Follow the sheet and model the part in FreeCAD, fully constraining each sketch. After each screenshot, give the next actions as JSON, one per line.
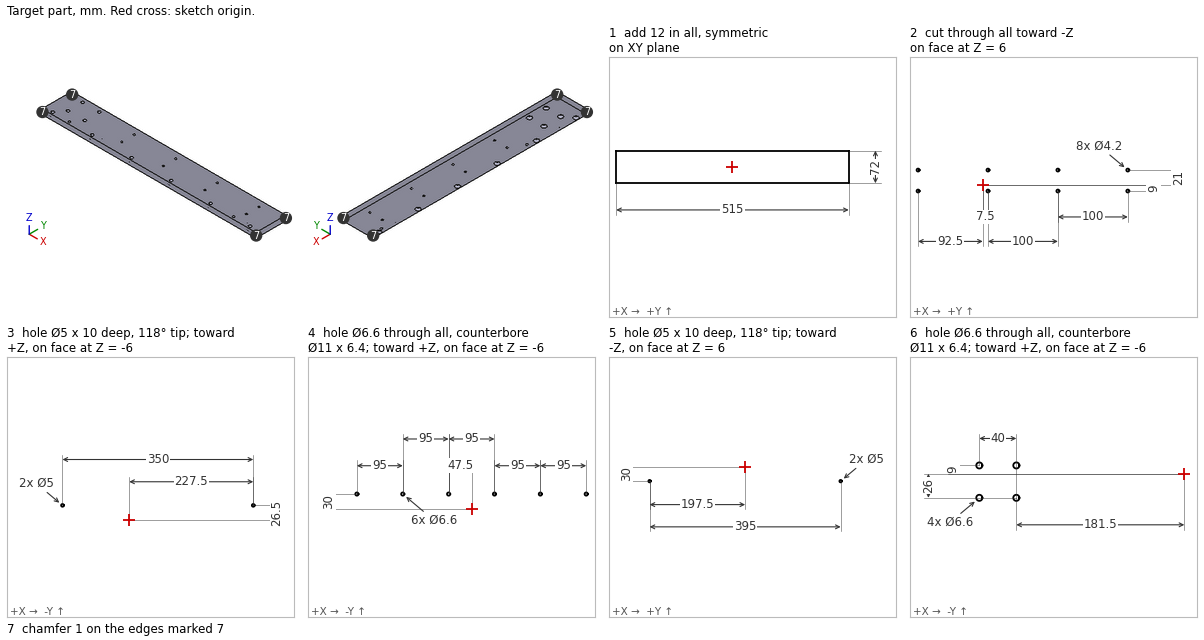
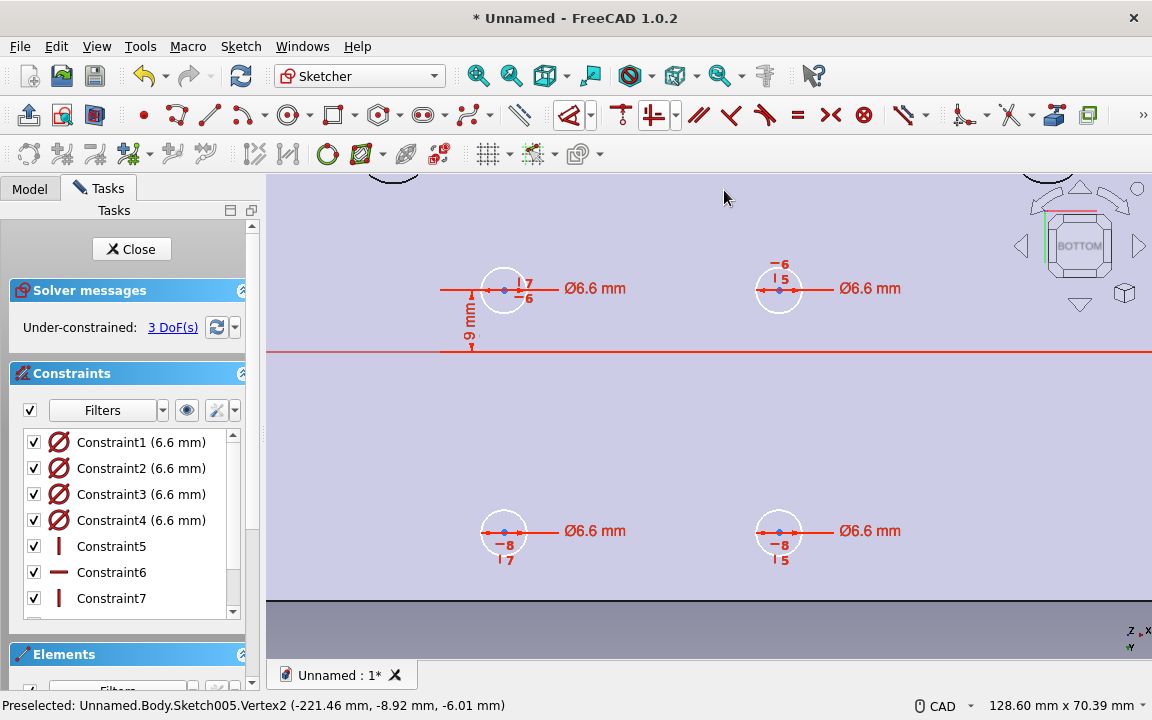
{"action": "left_click", "coordinate": [779, 533]}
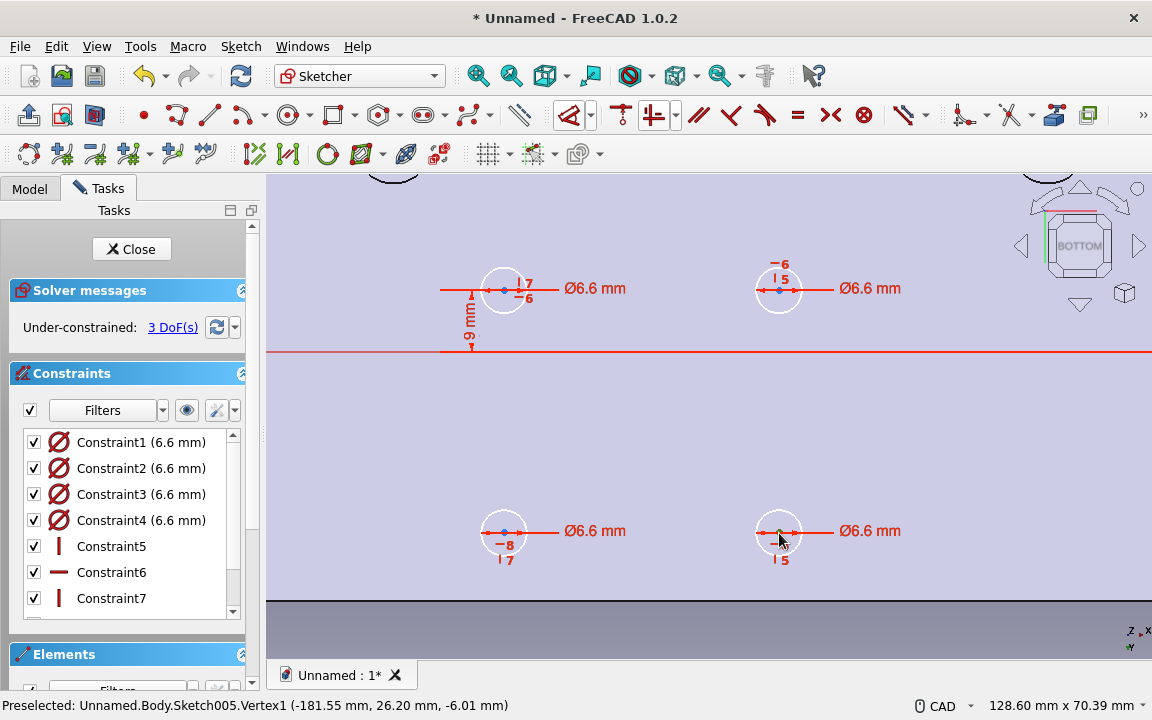
{"action": "left_click", "coordinate": [590, 116]}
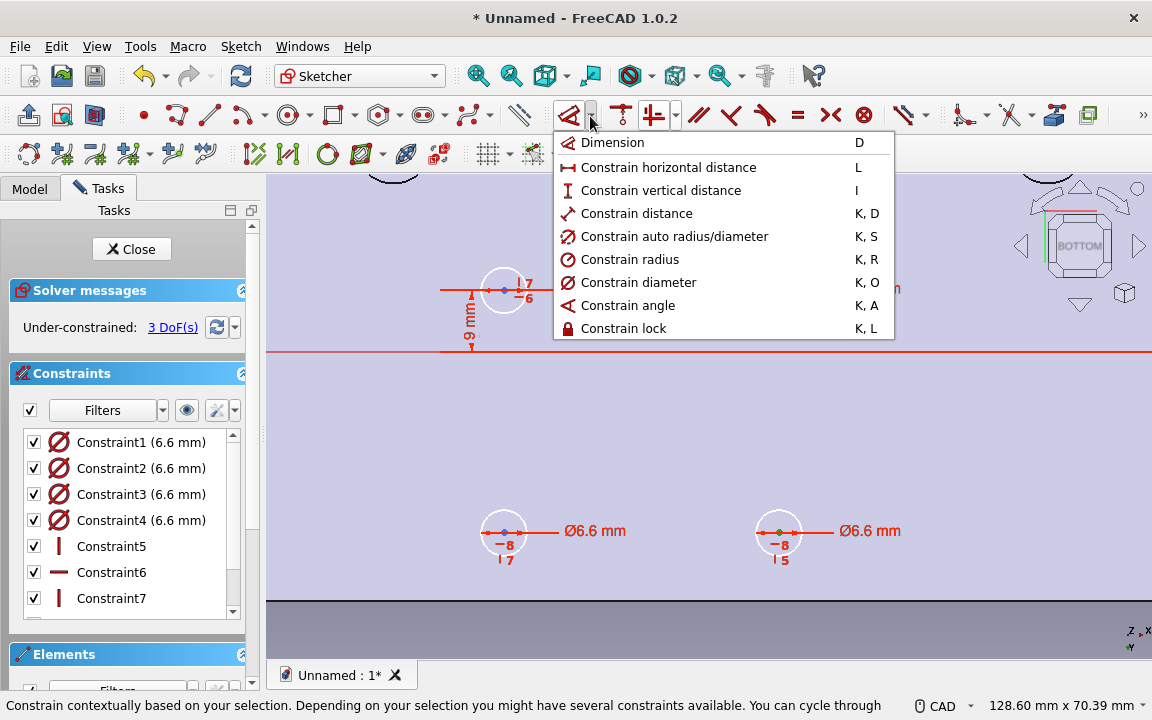
{"action": "left_click", "coordinate": [724, 190]}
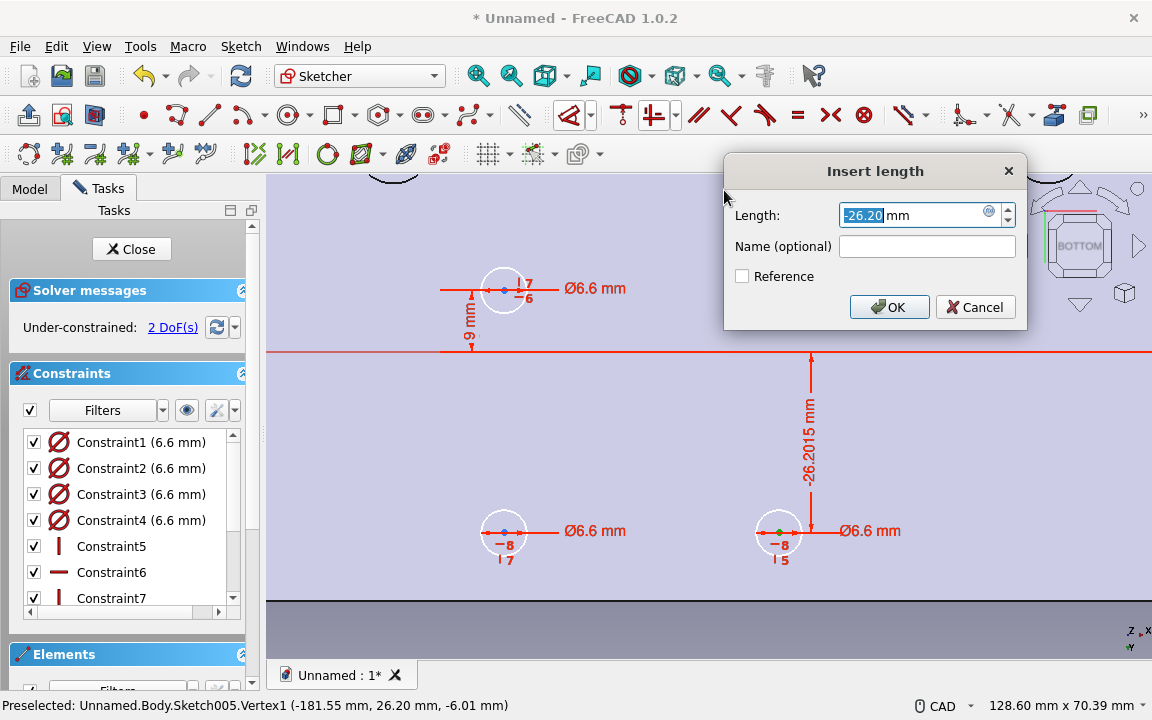
{"action": "type", "text": "-26"}
{"action": "key", "text": "Return"}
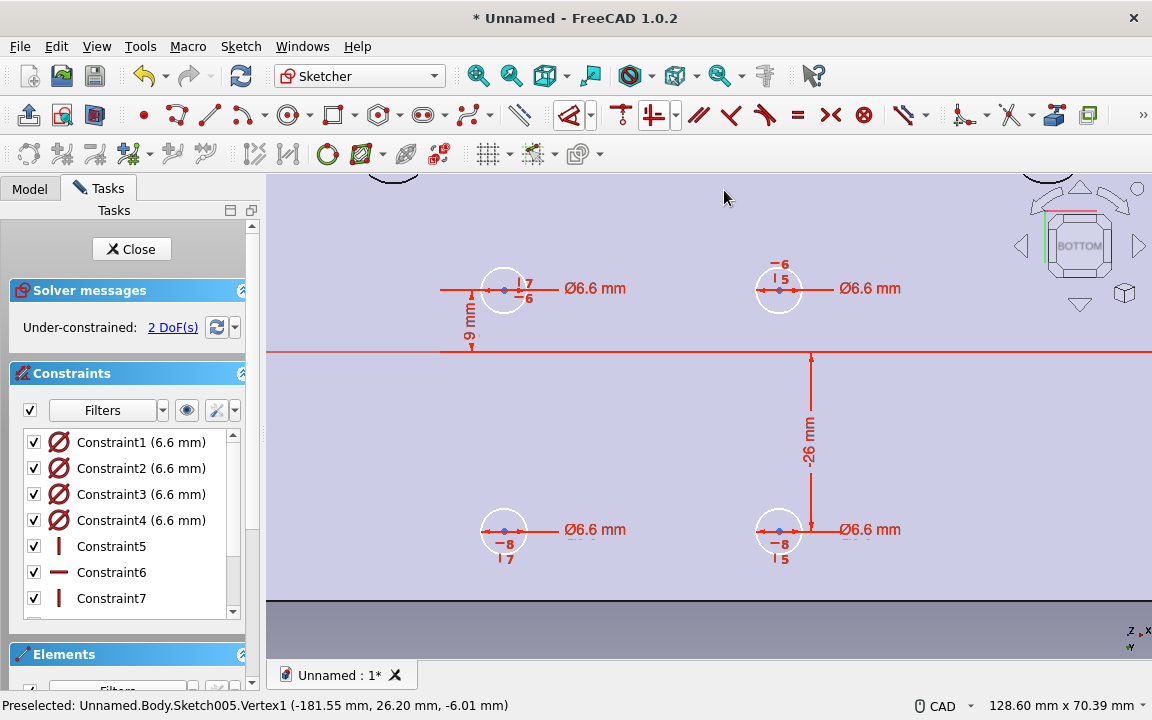
{"action": "left_click", "coordinate": [779, 532]}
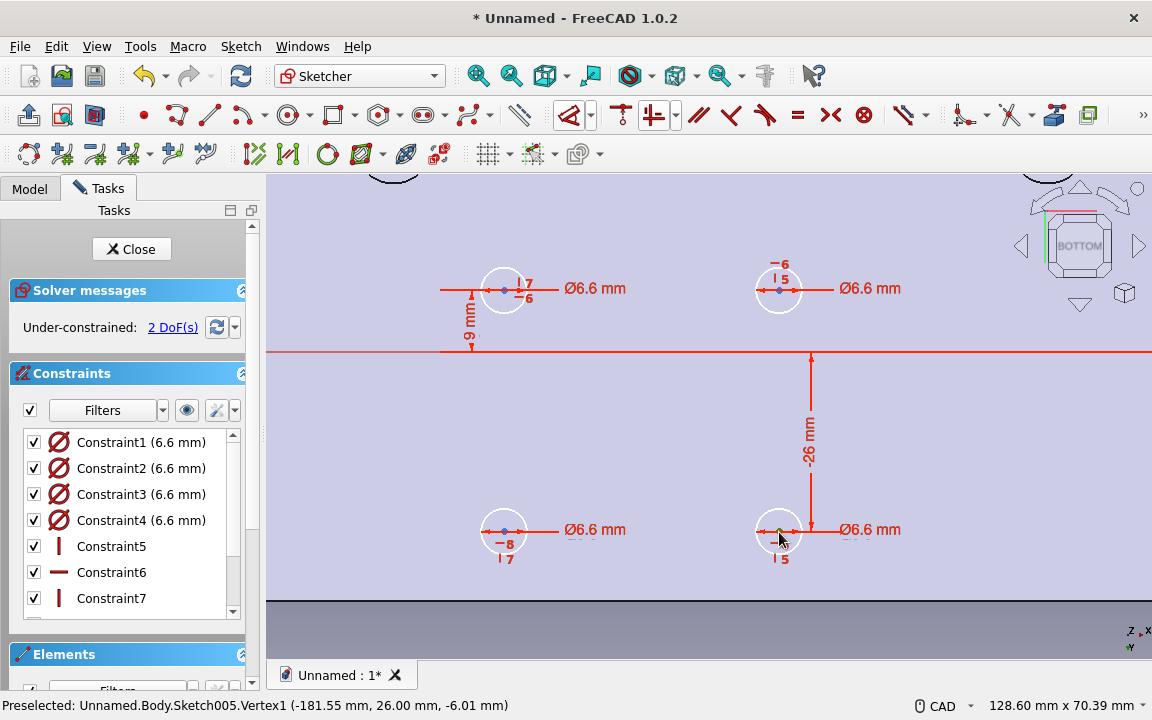
{"action": "left_click", "coordinate": [504, 290]}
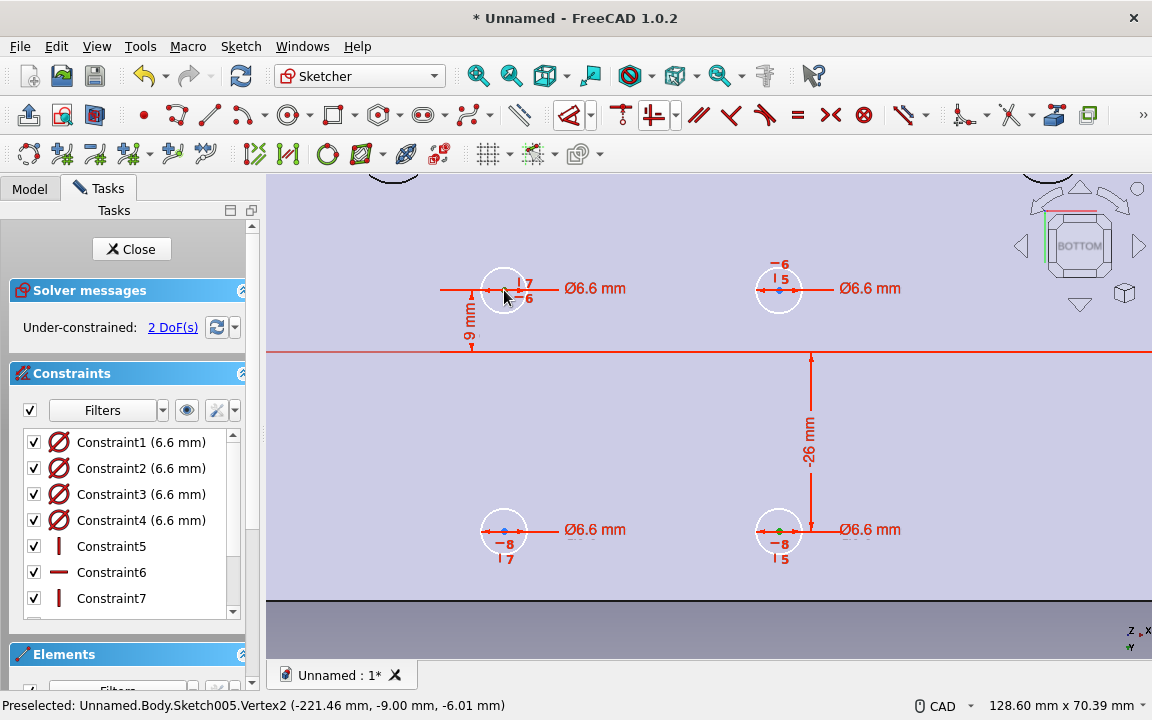
{"action": "left_click", "coordinate": [590, 116]}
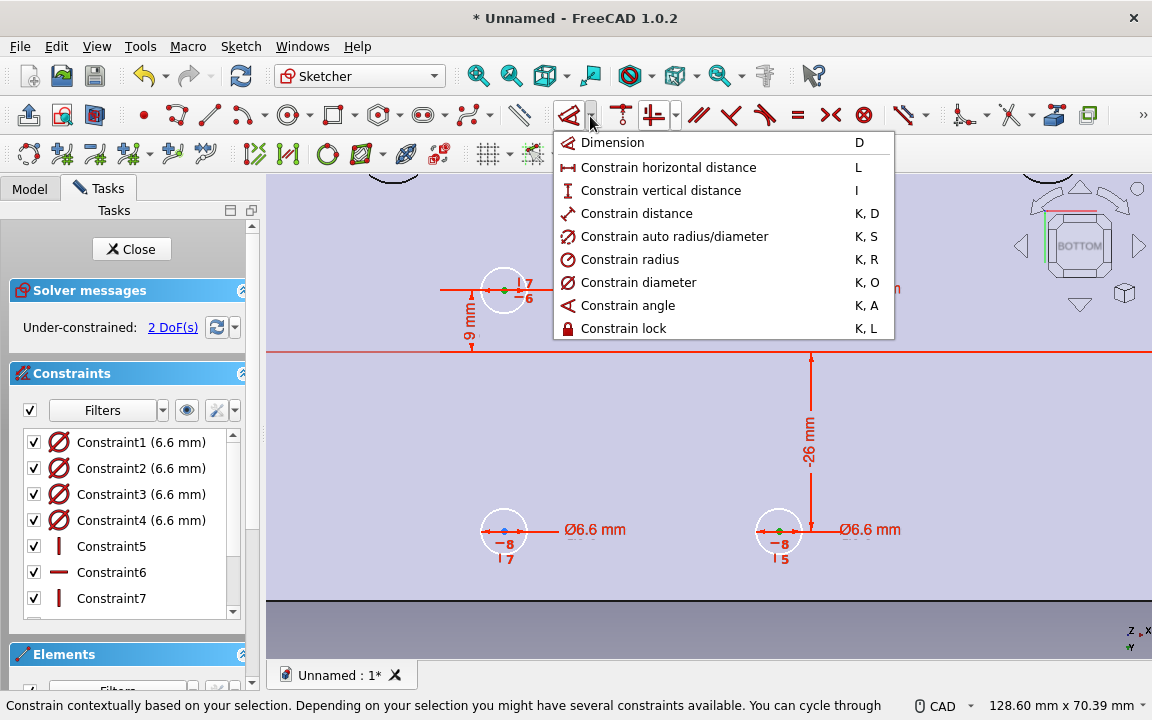
{"action": "left_click", "coordinate": [724, 168]}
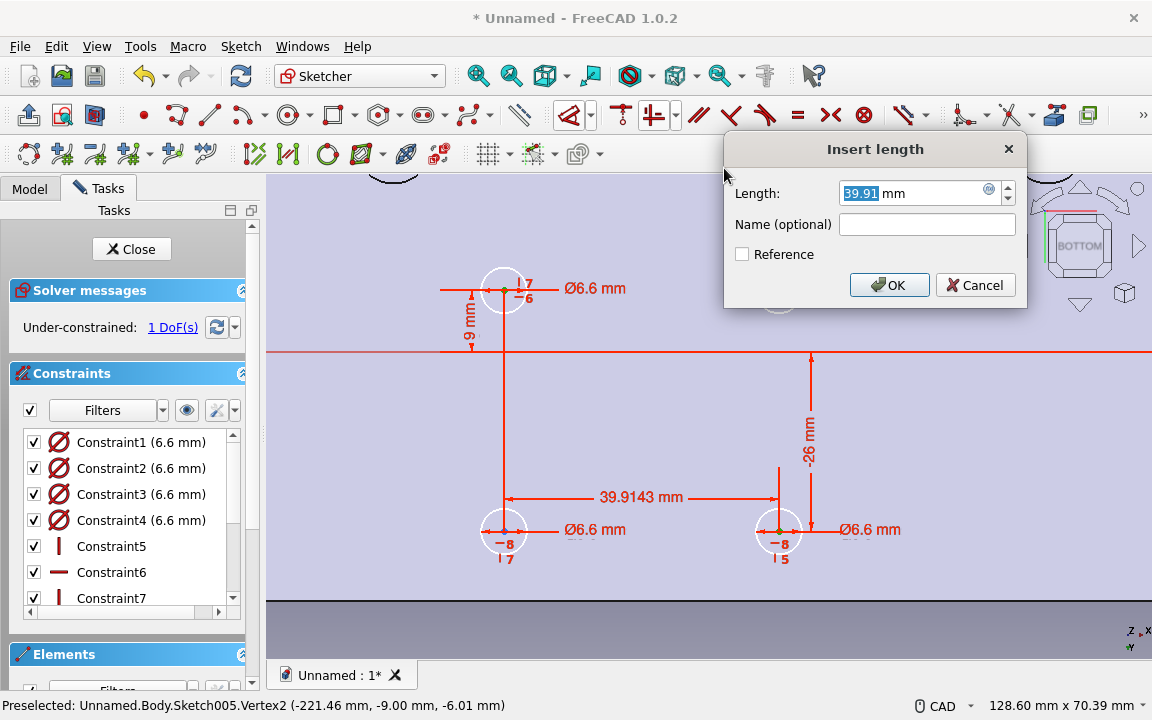
{"action": "type", "text": "40"}
{"action": "key", "text": "Return"}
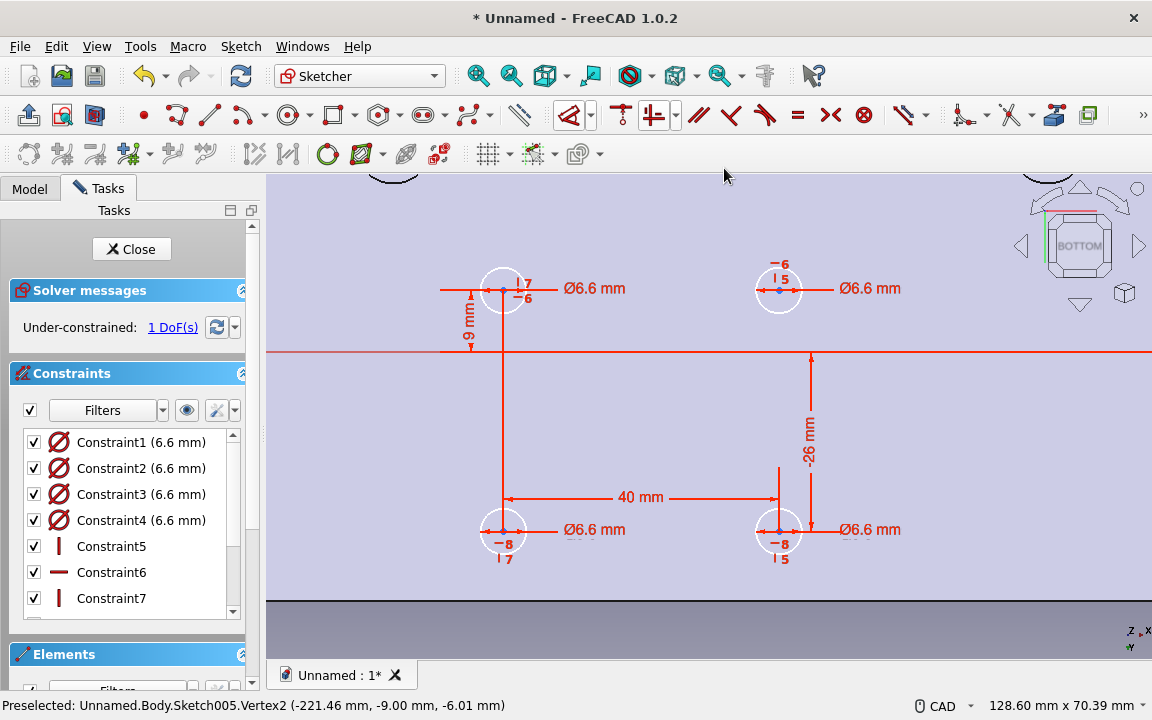
{"action": "left_click", "coordinate": [779, 532]}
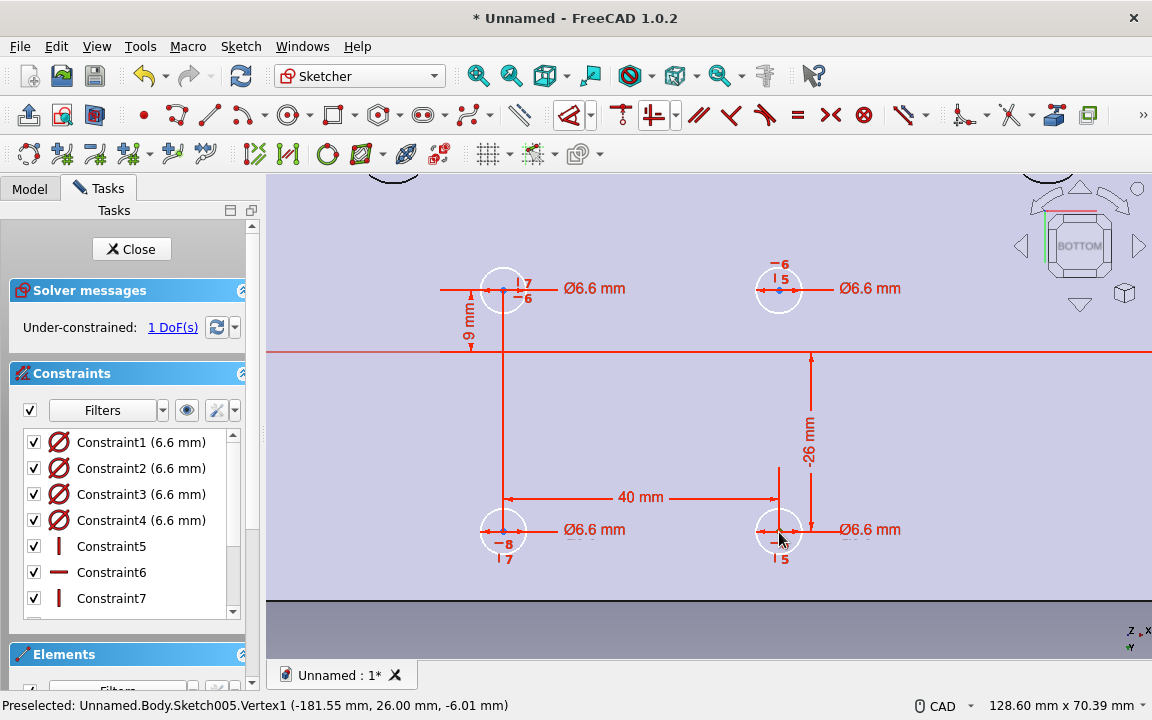
{"action": "key", "text": "l"}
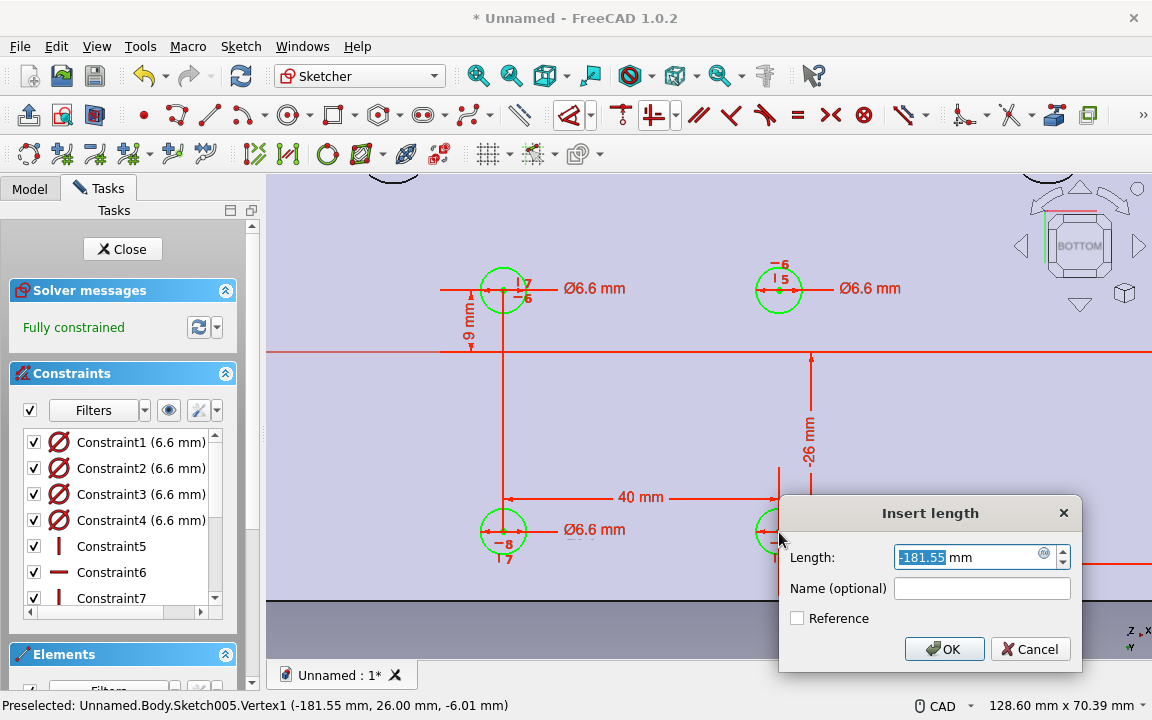
{"action": "type", "text": "-181.5"}
{"action": "key", "text": "Return"}